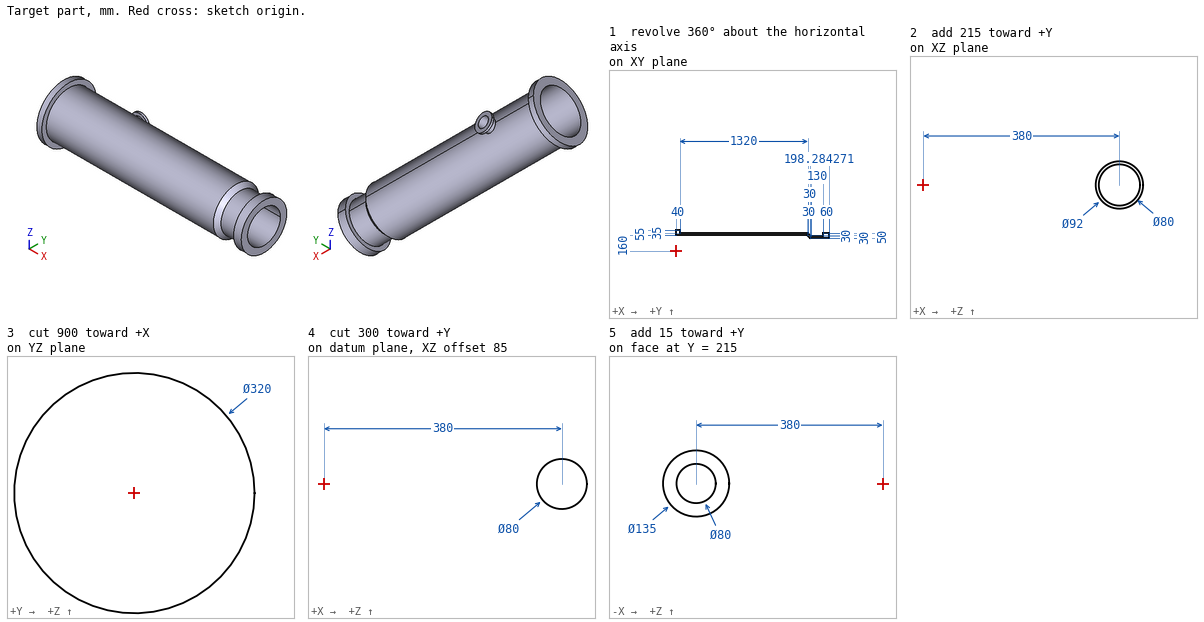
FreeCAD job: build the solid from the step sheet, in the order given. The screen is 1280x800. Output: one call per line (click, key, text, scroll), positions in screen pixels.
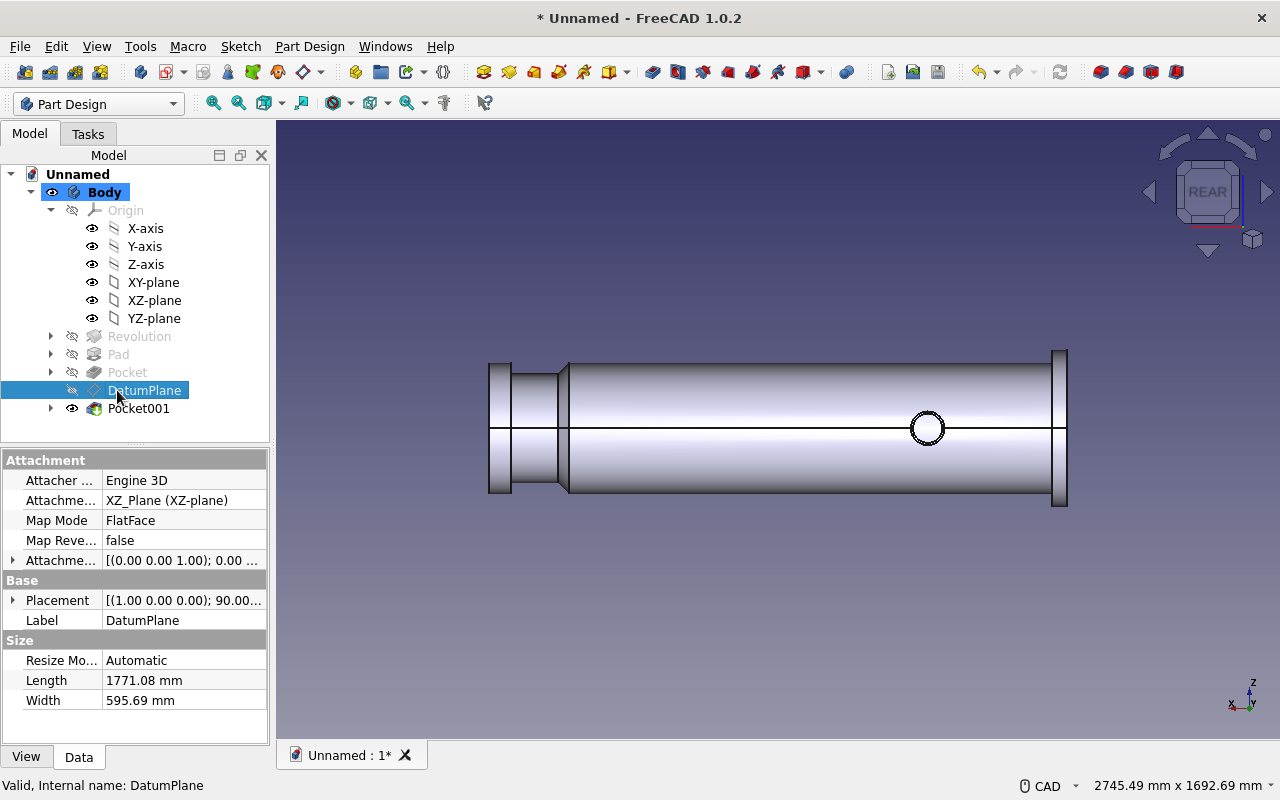
scroll(923, 413, up, 15)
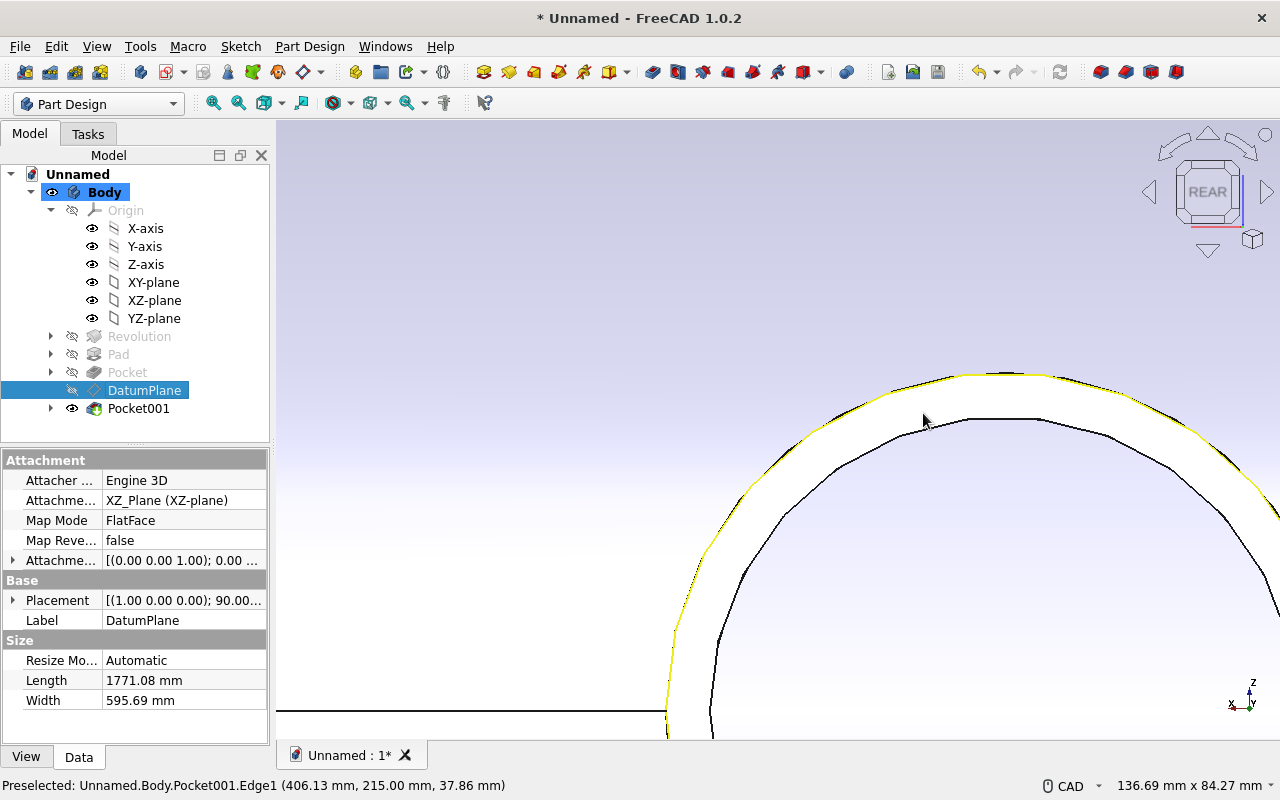
click(907, 420)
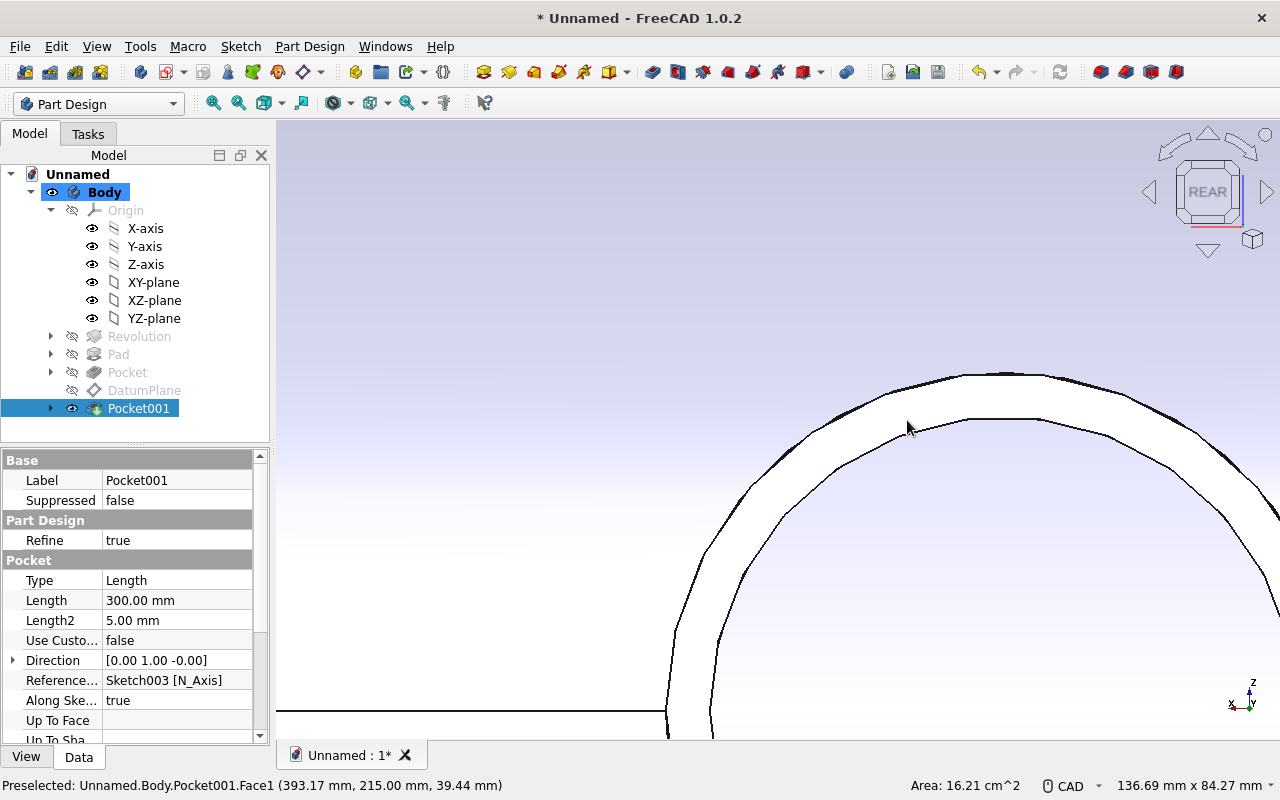
click(166, 72)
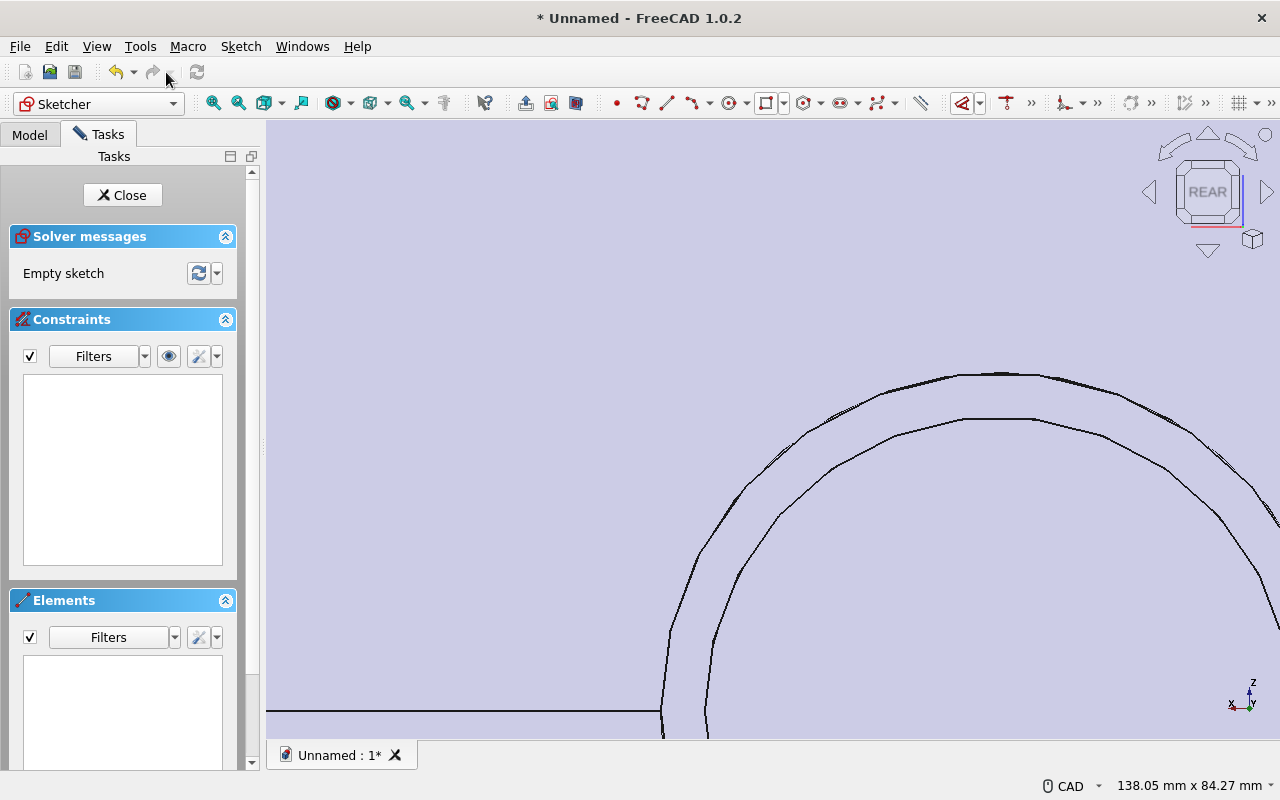
scroll(533, 266, down, 5)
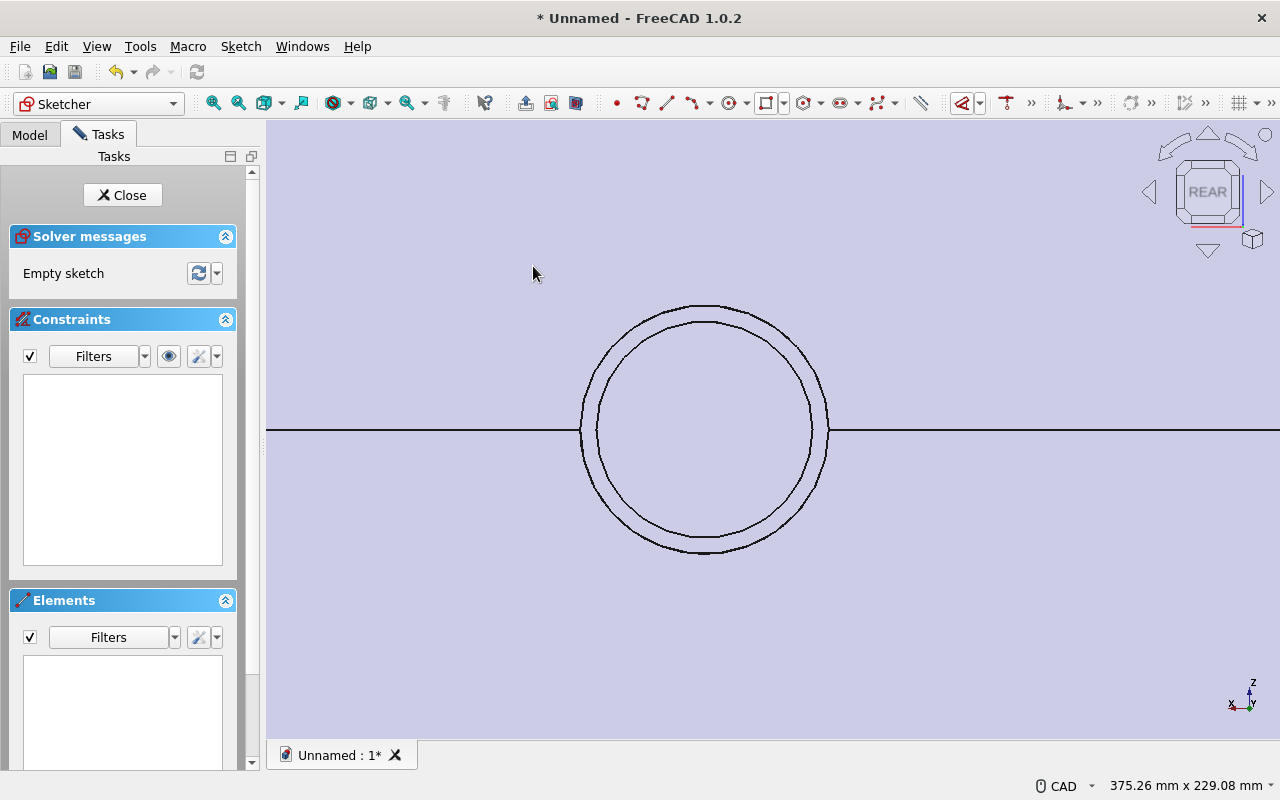
key(g)
key(c)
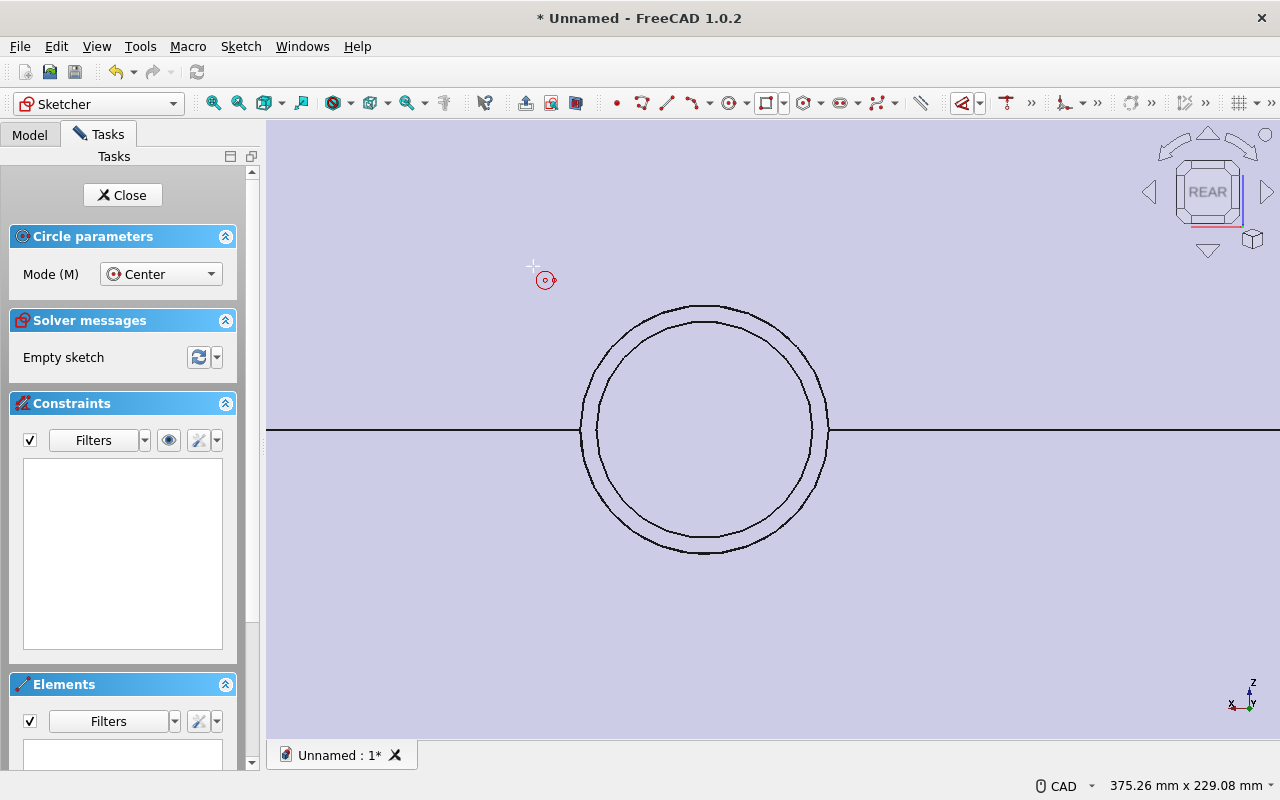
click(704, 430)
move(833, 301)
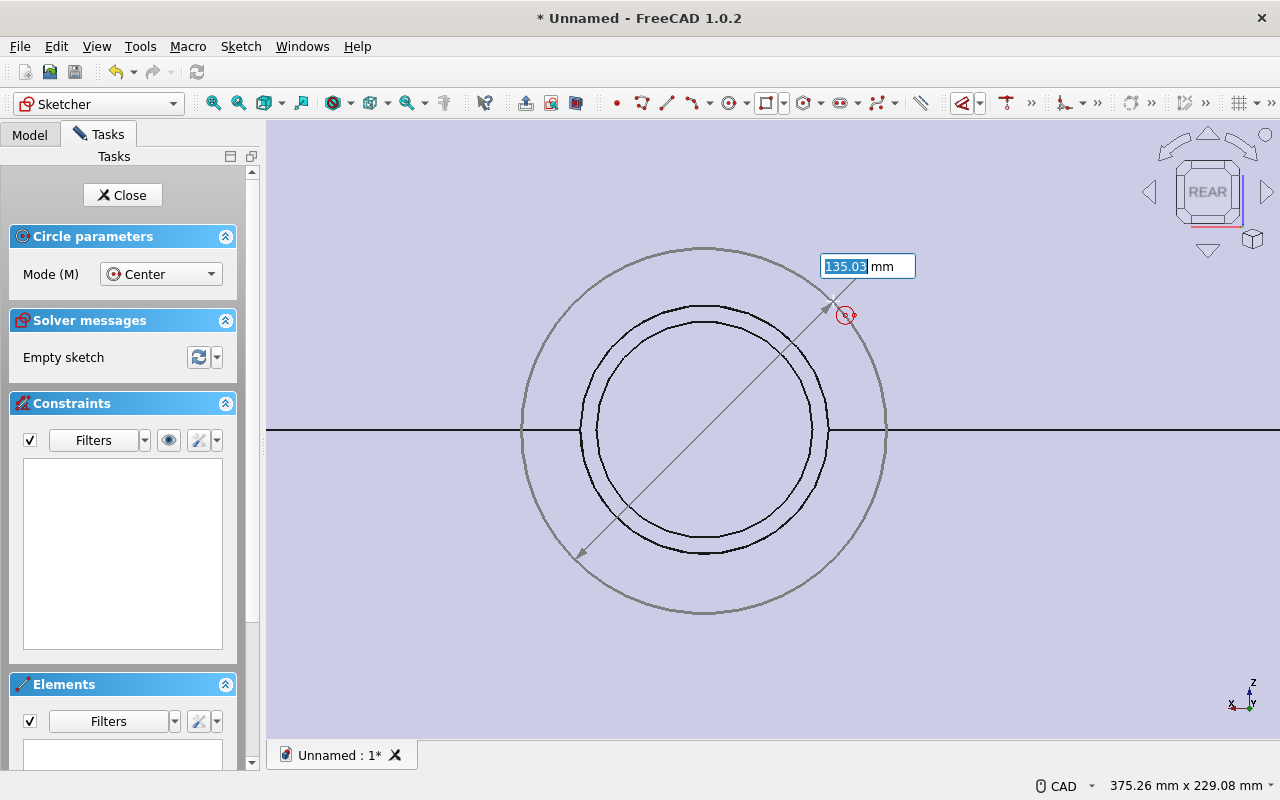
text(135)
key(Return)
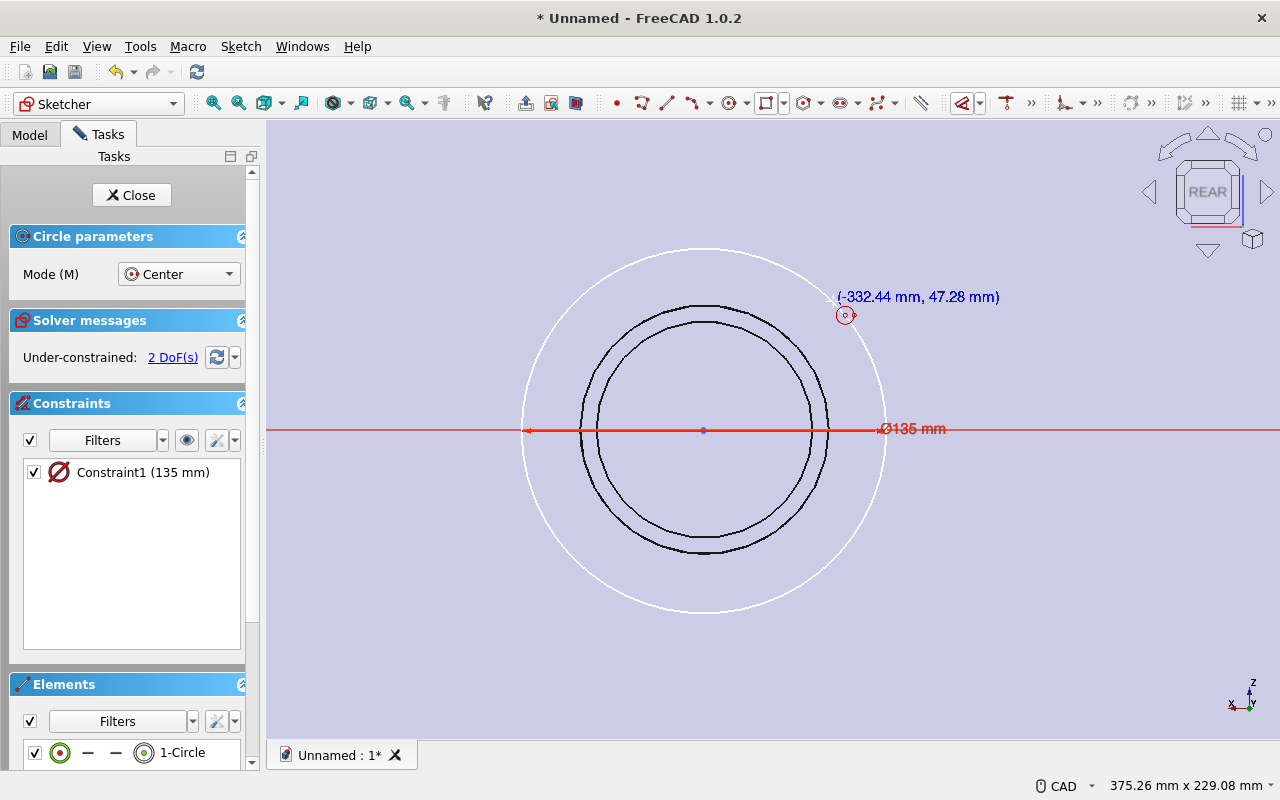
click(704, 431)
move(781, 353)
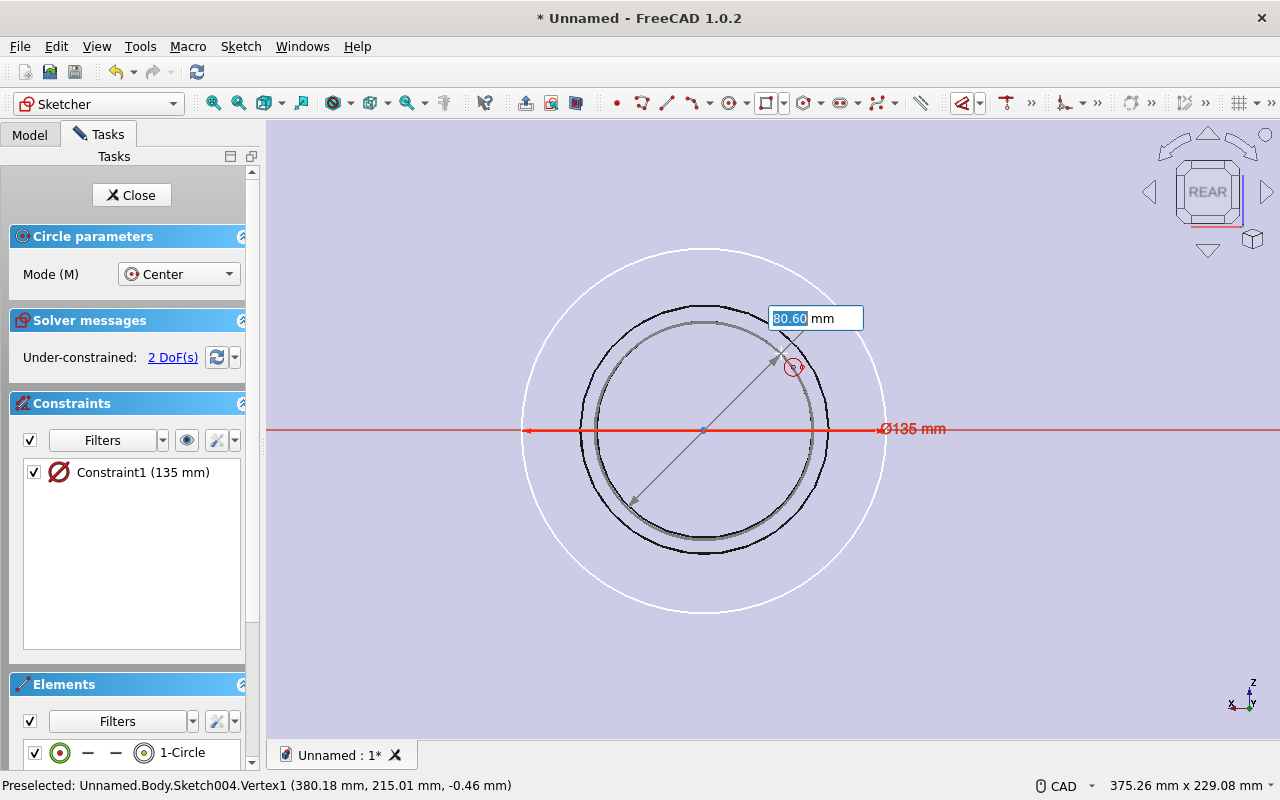
text(80)
key(Return)
key(Escape)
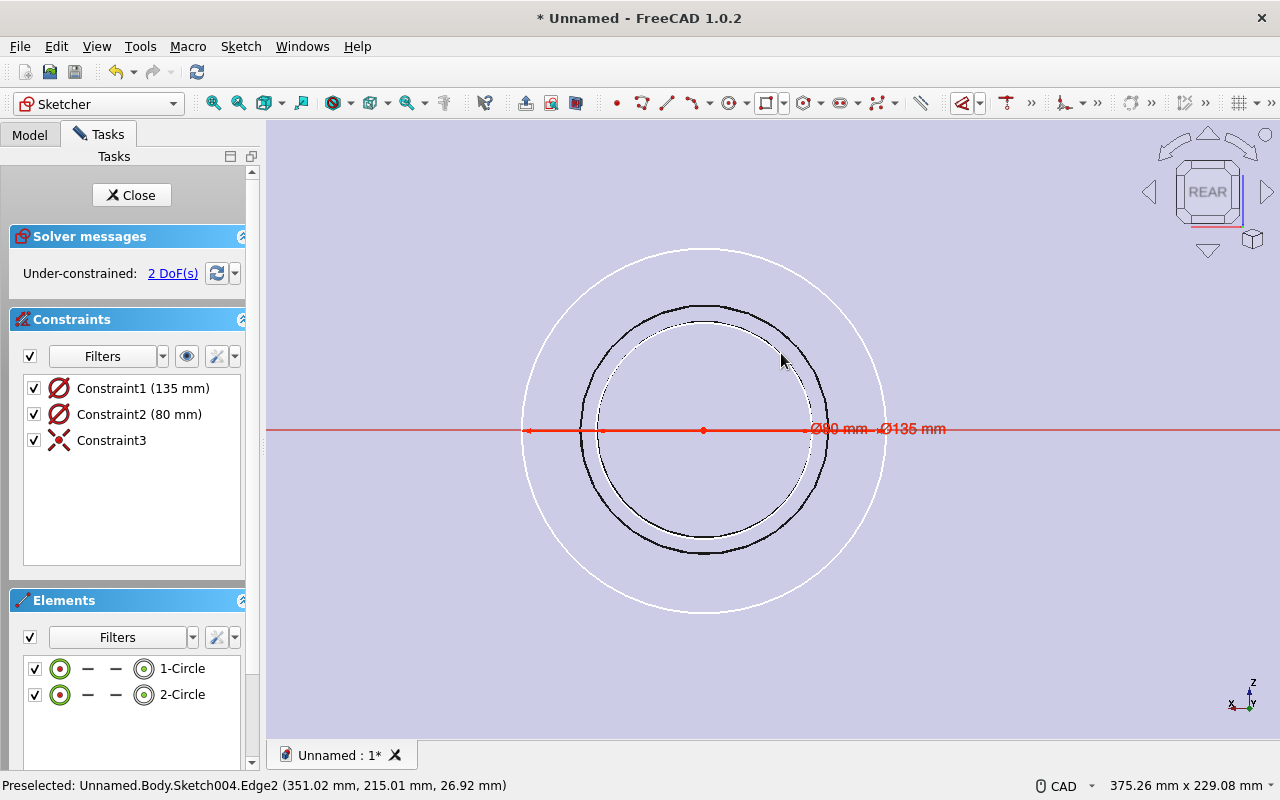
click(704, 431)